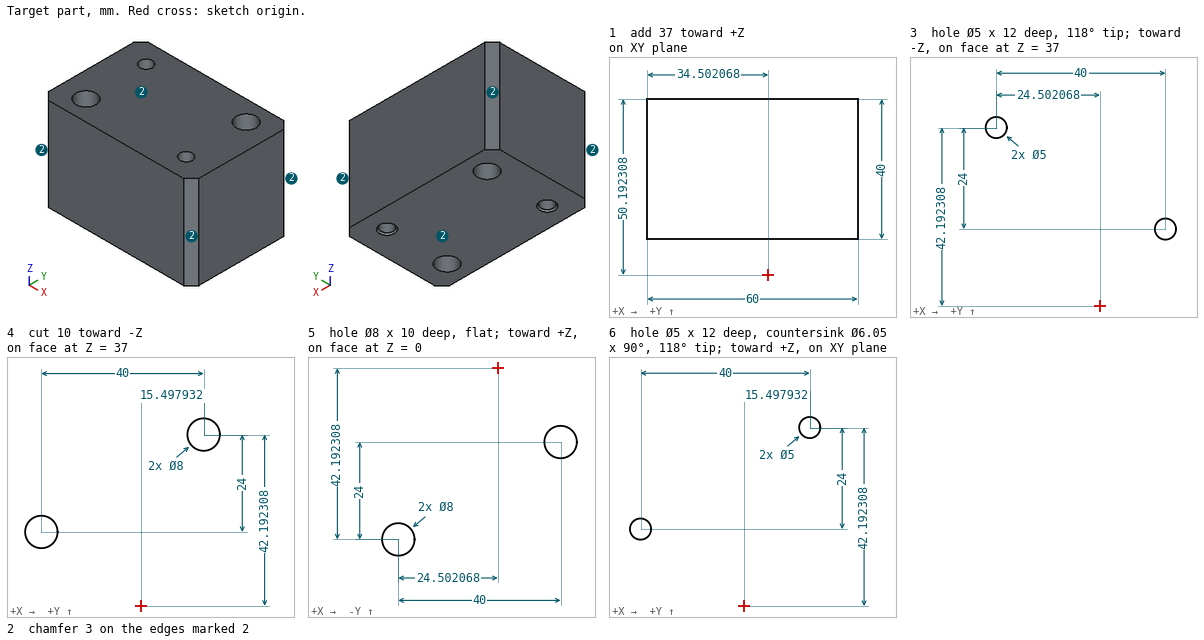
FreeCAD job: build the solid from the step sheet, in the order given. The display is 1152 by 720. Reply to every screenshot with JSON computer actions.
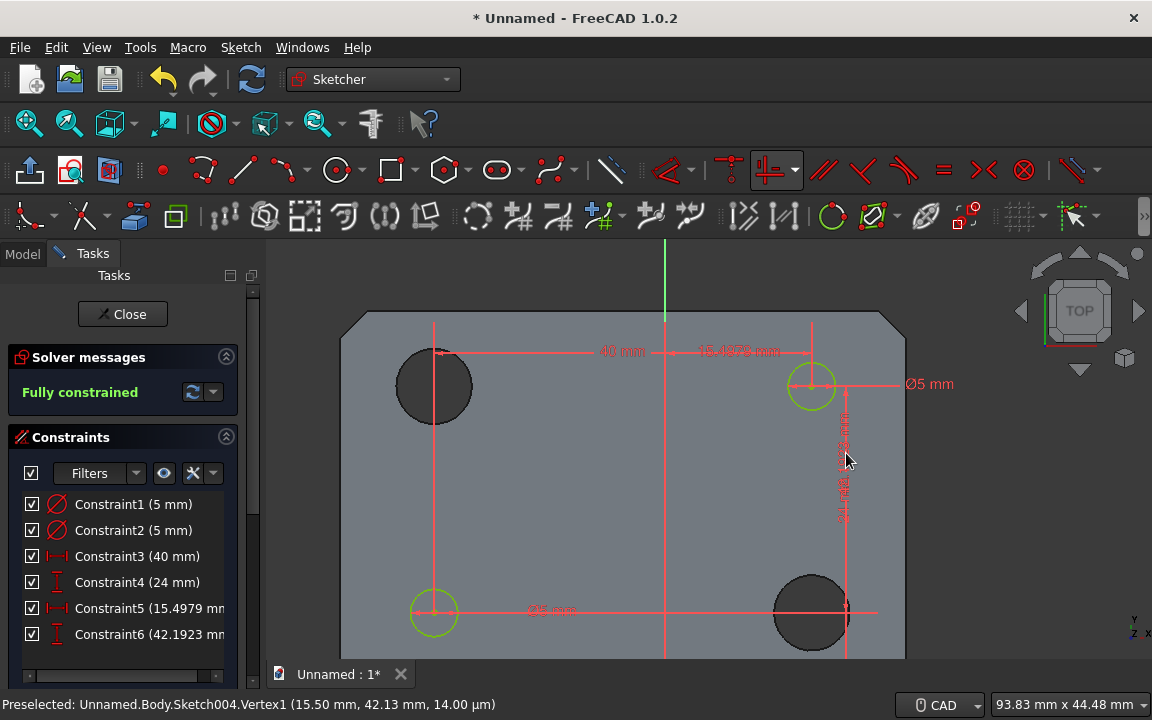
{"action": "left_click", "coordinate": [123, 314]}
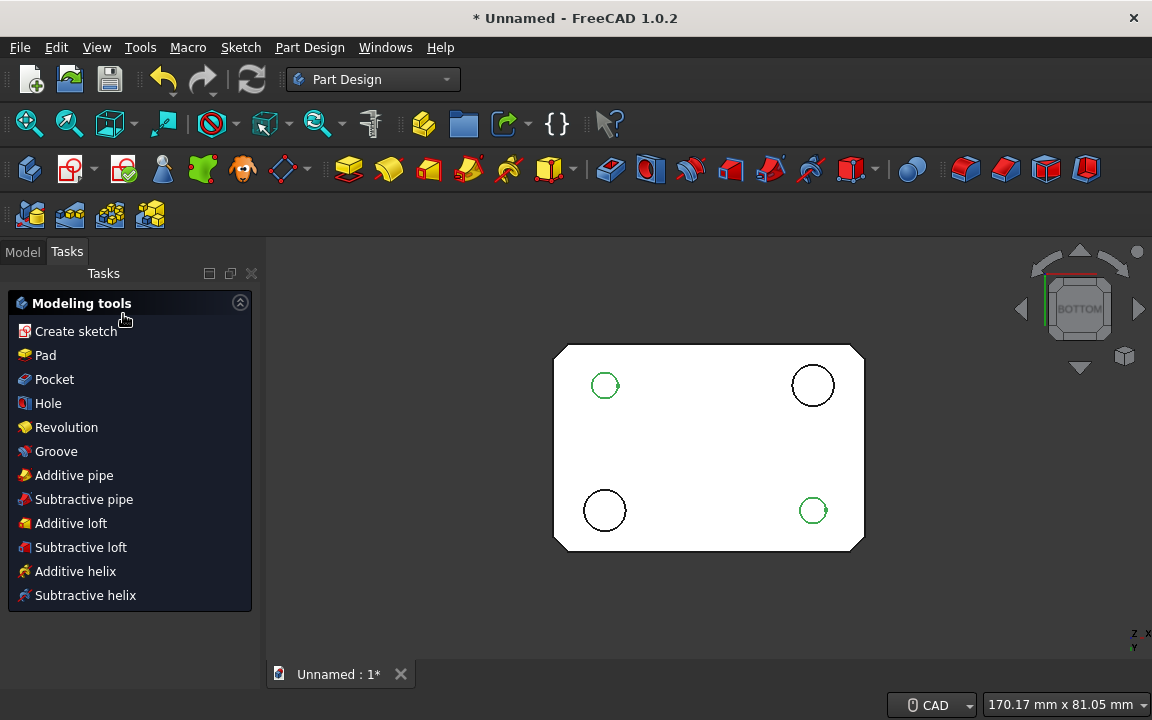
{"action": "left_click", "coordinate": [652, 170]}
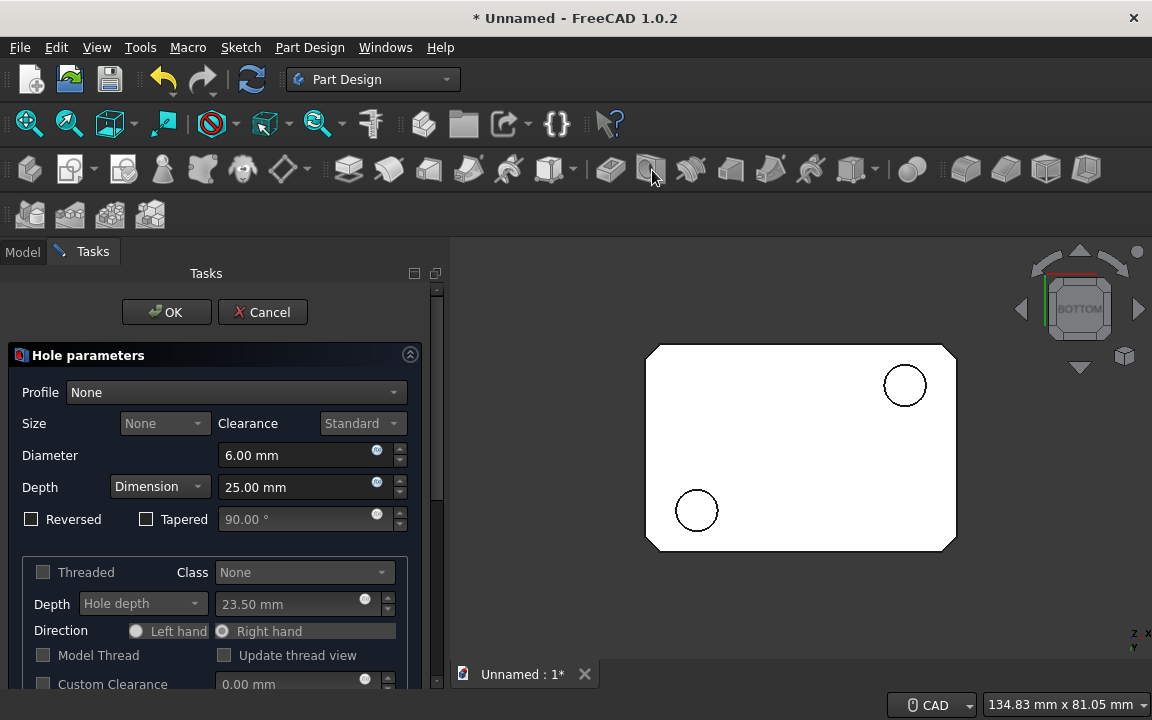
{"action": "triple_click", "coordinate": [305, 455]}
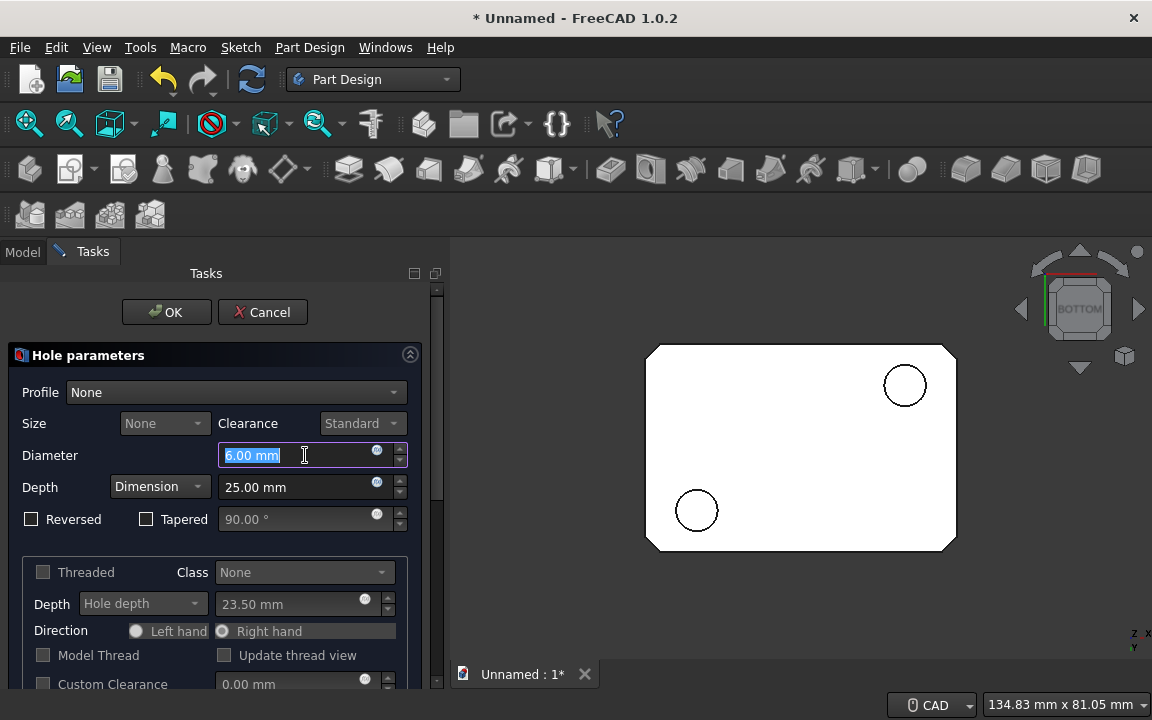
{"action": "type", "text": "5"}
{"action": "key", "text": "Tab"}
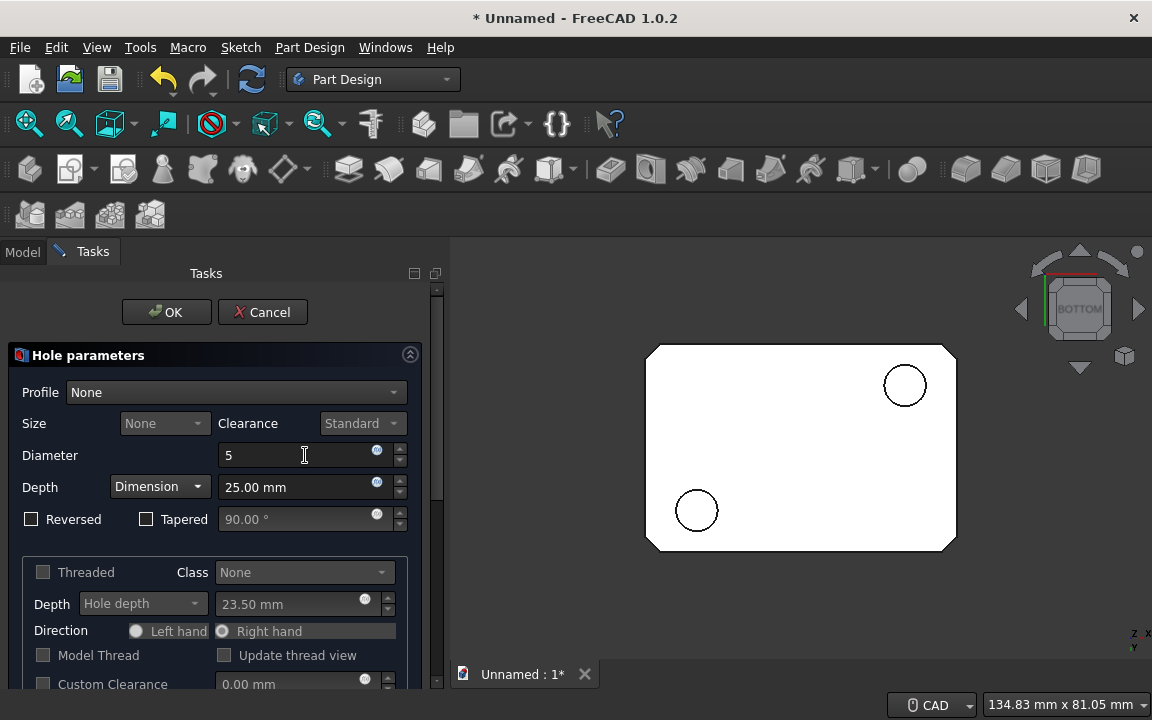
{"action": "triple_click", "coordinate": [305, 487]}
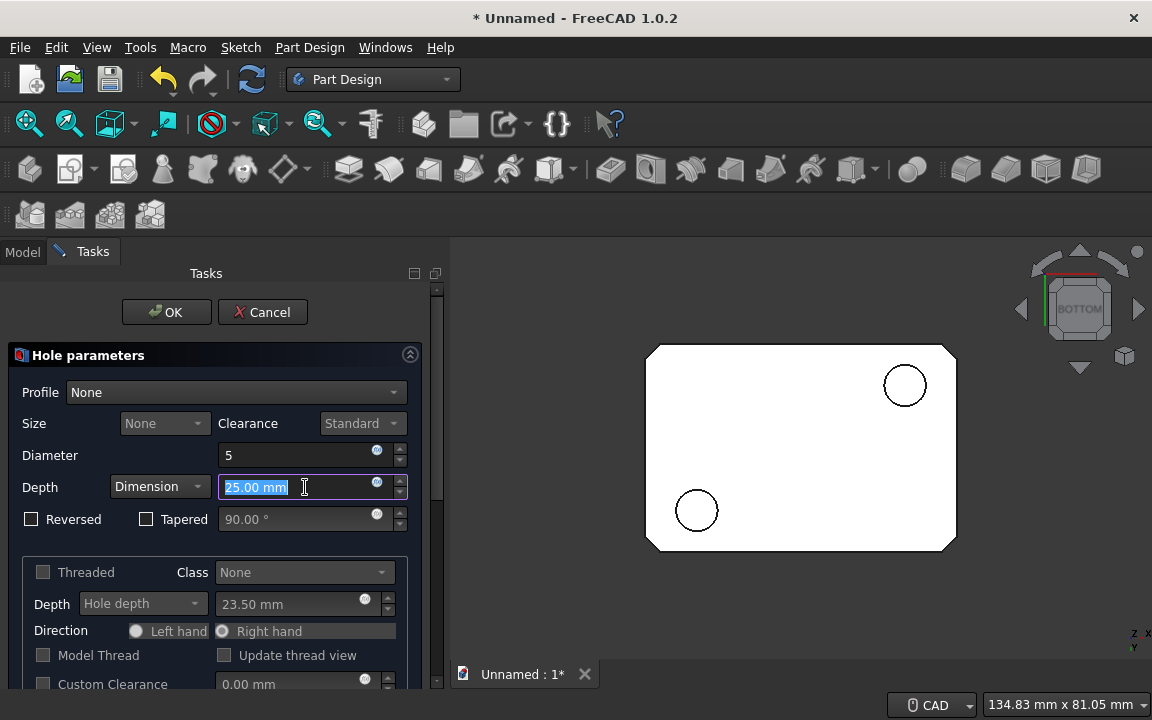
{"action": "type", "text": "12"}
{"action": "key", "text": "Tab"}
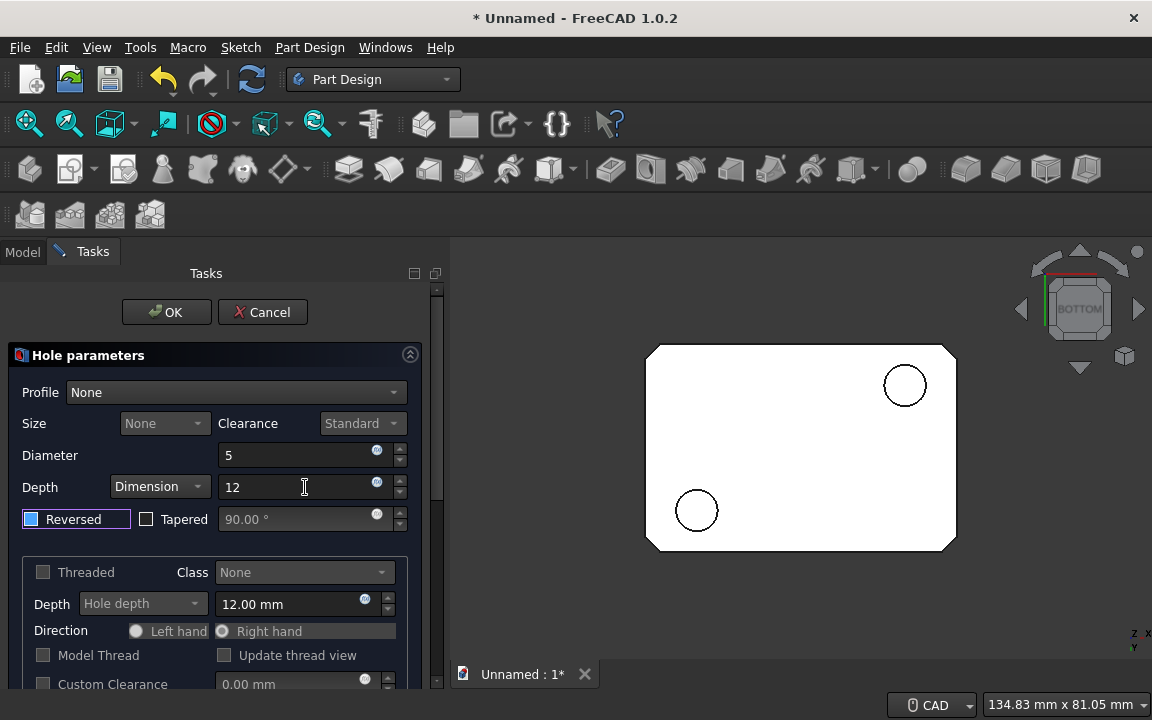
{"action": "left_click", "coordinate": [30, 519]}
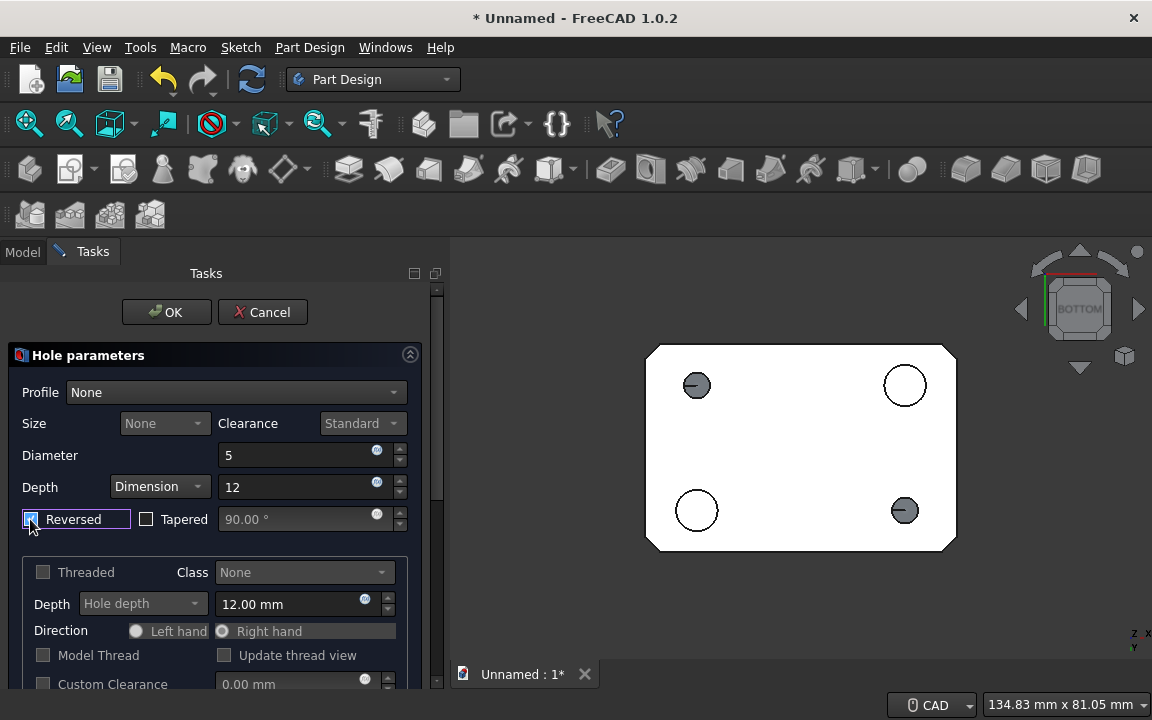
{"action": "scroll", "coordinate": [437, 486], "scroll_direction": "down", "scroll_amount": 3}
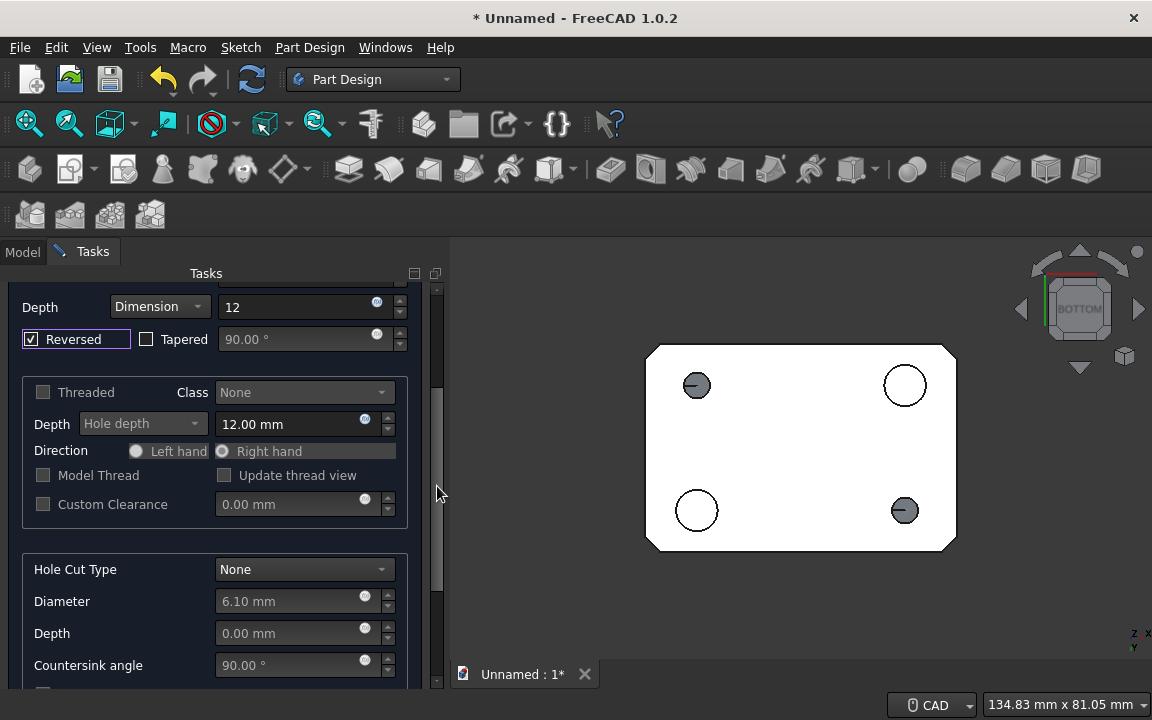
{"action": "left_click", "coordinate": [306, 570]}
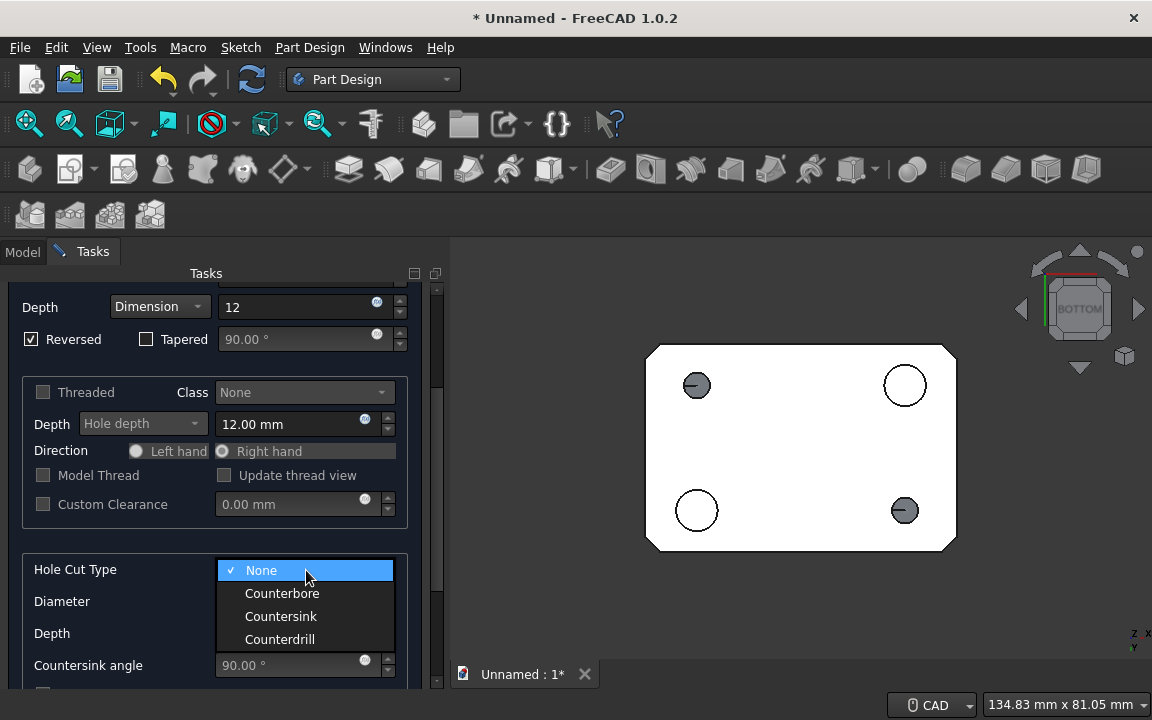
{"action": "left_click", "coordinate": [304, 616]}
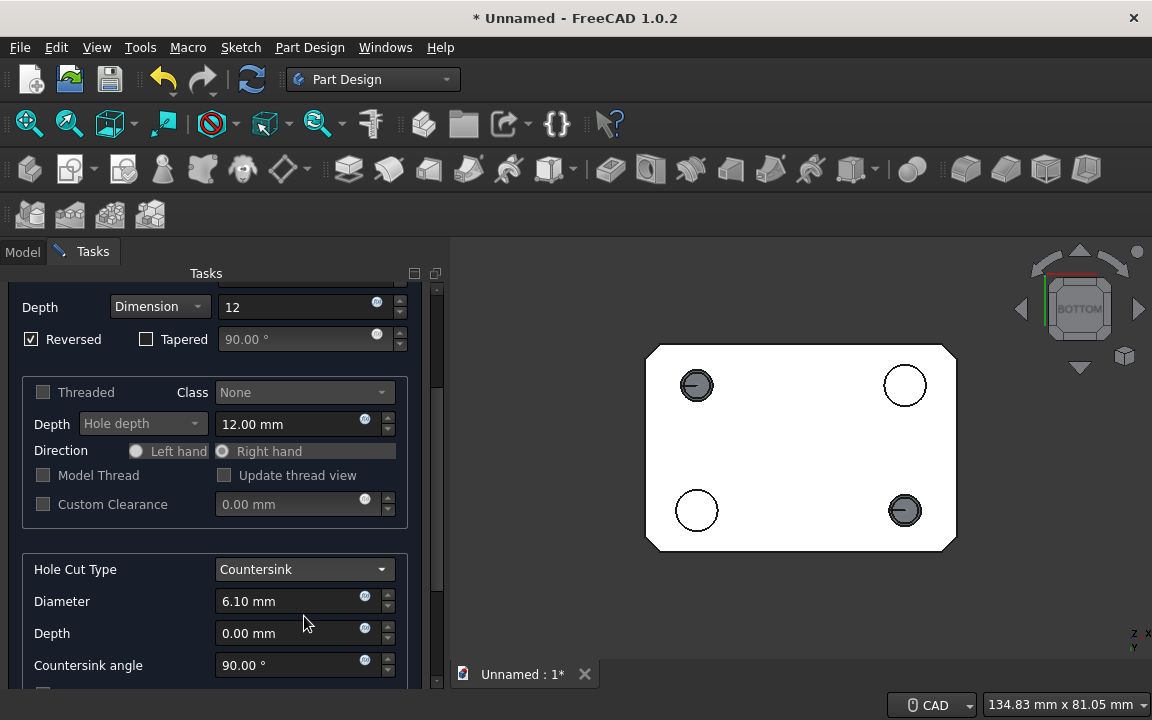
{"action": "triple_click", "coordinate": [298, 601]}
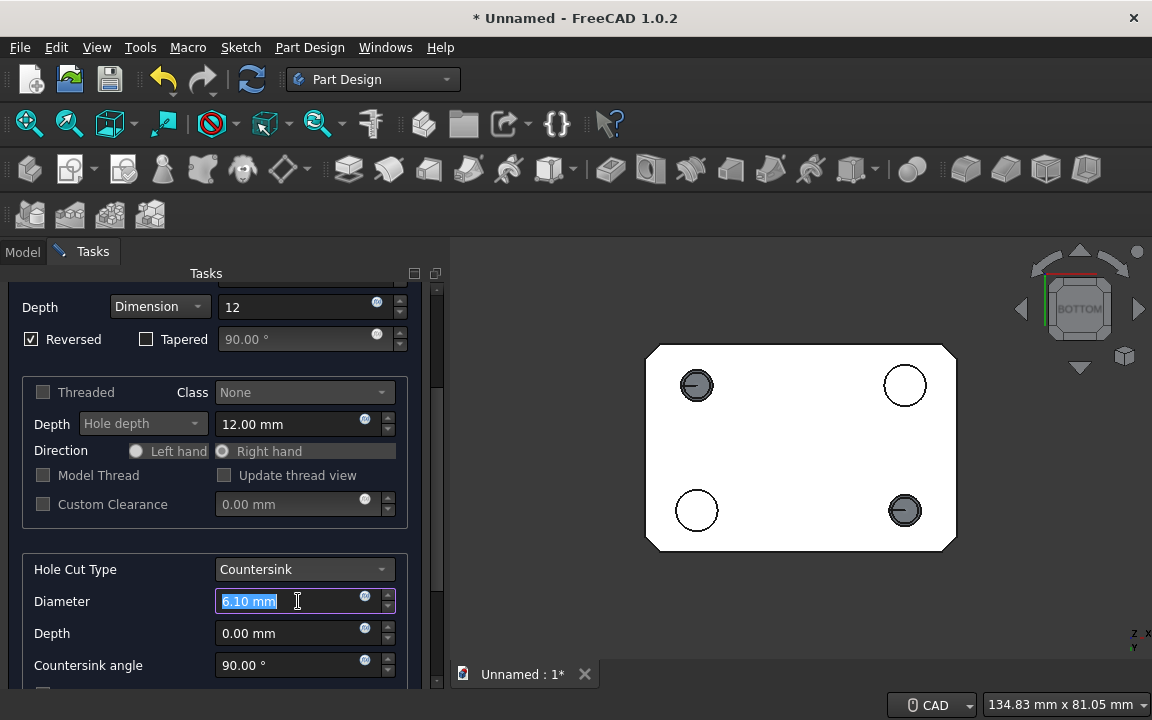
{"action": "type", "text": "6.05"}
{"action": "key", "text": "Tab"}